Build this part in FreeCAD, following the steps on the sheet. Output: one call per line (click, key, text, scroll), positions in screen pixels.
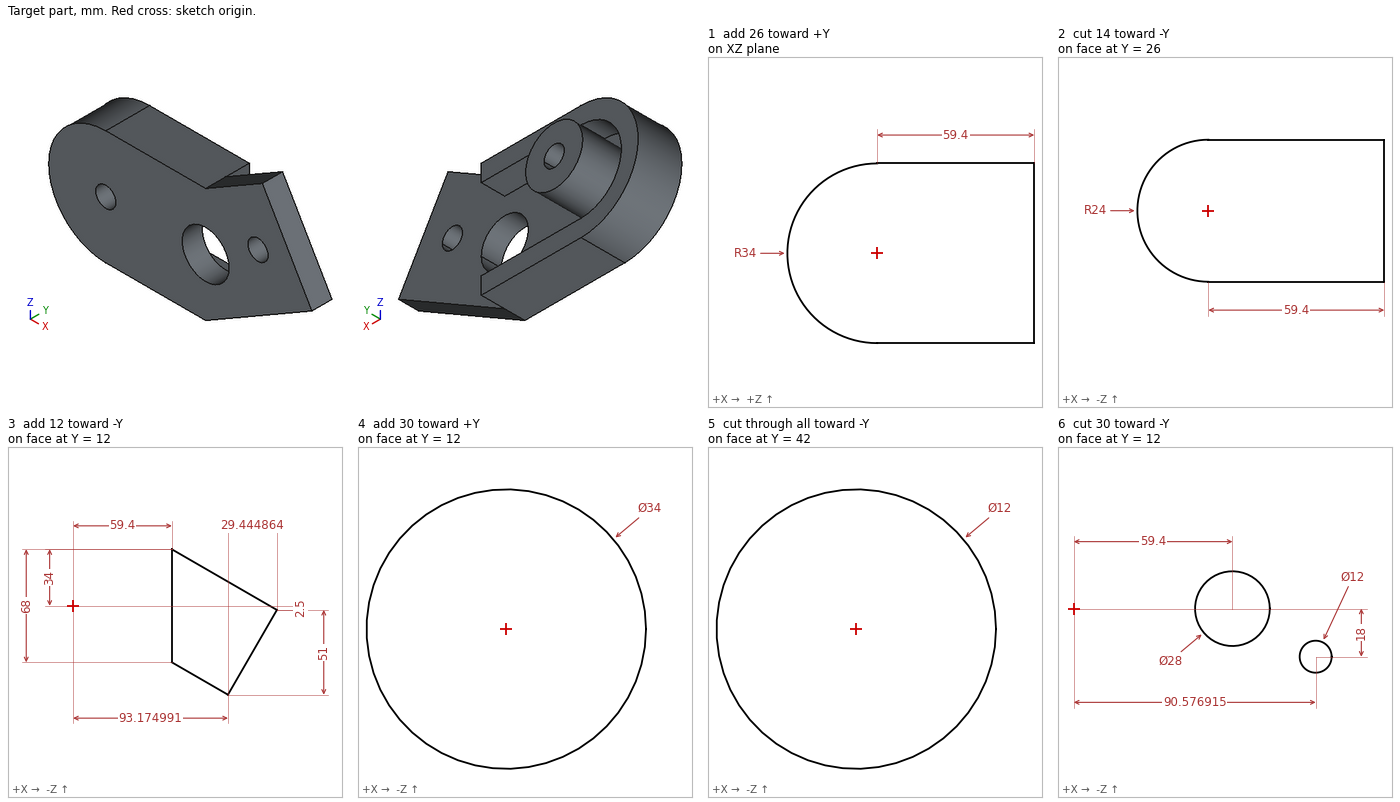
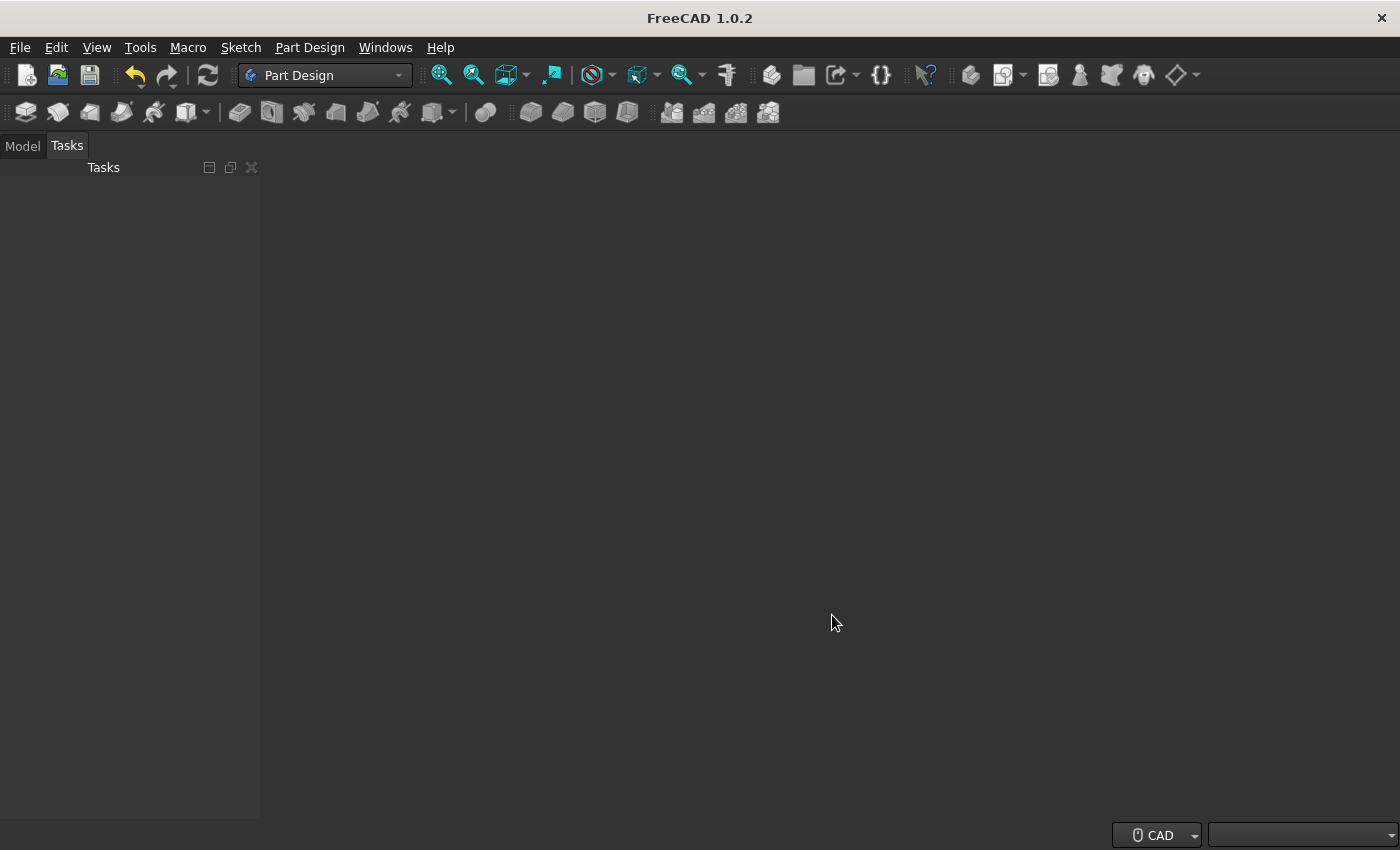
click(26, 76)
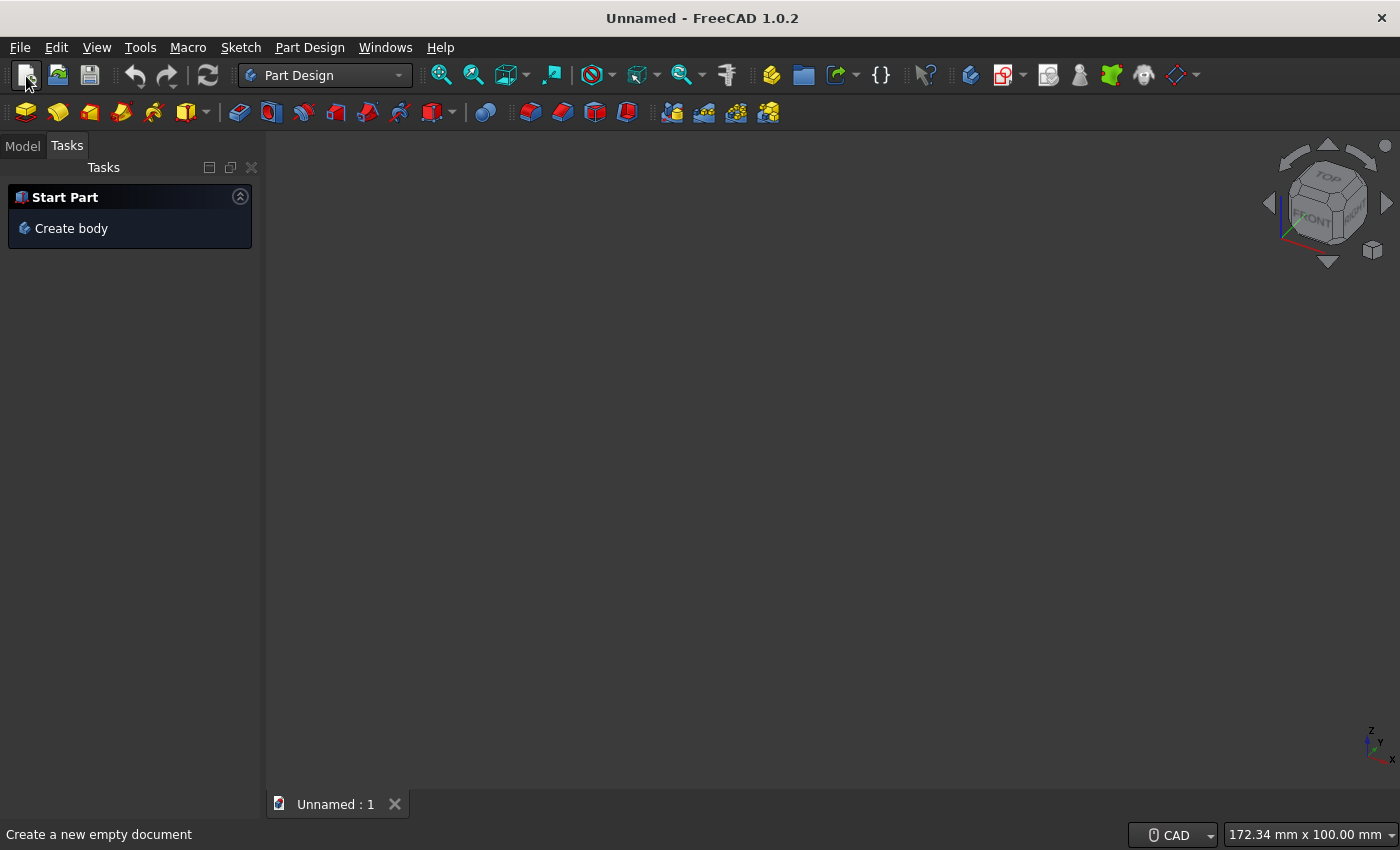
click(1004, 76)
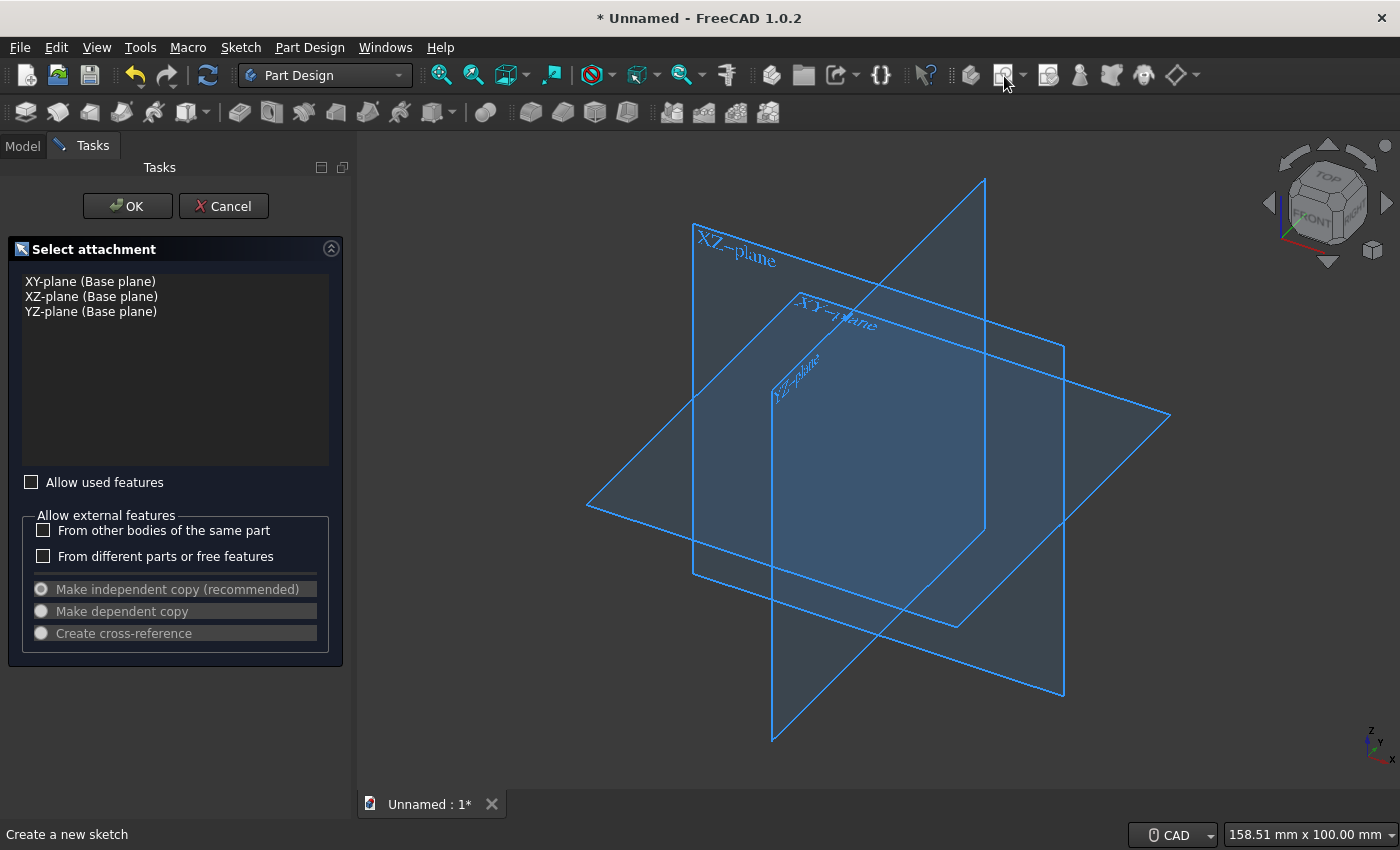
click(82, 296)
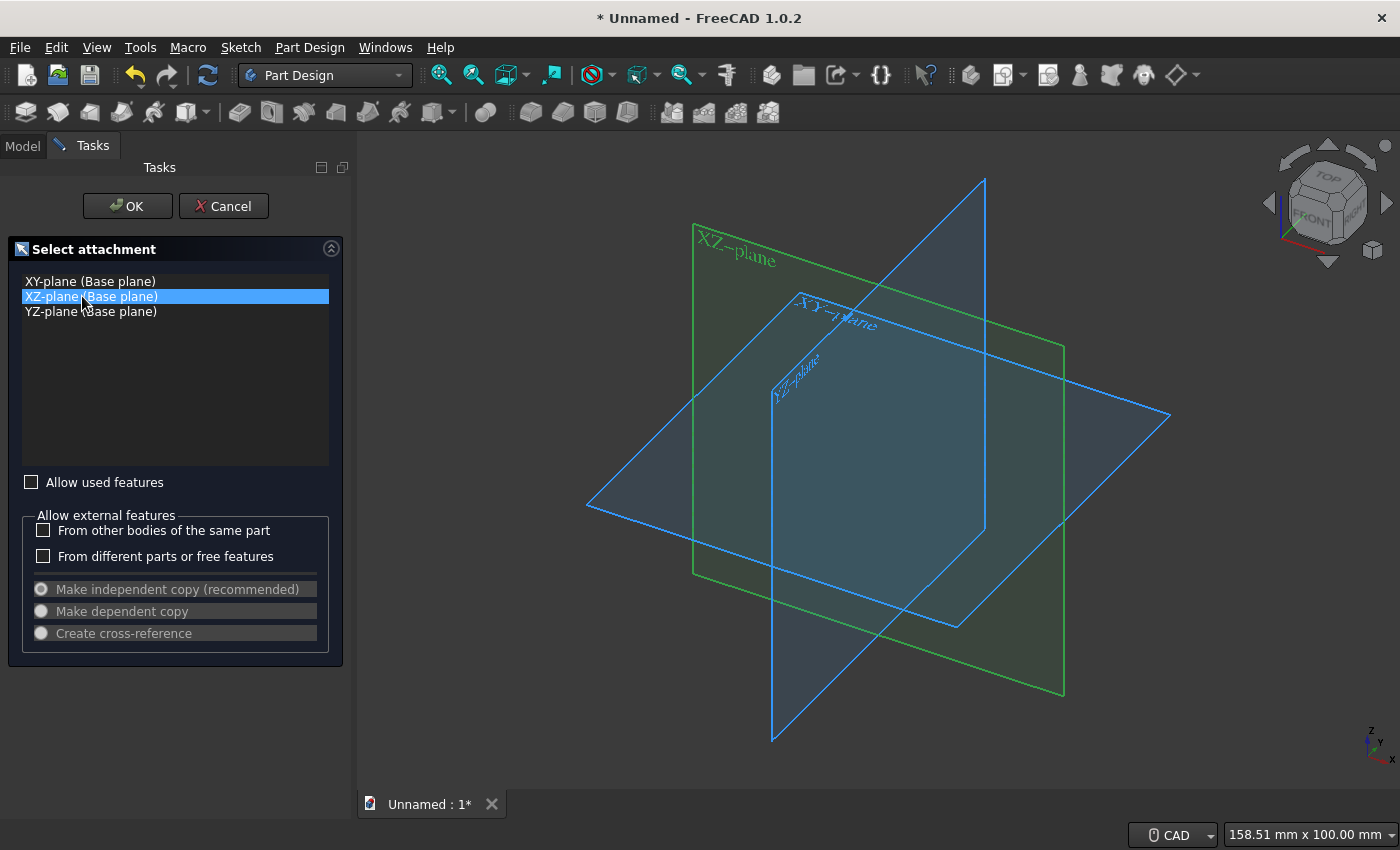
click(128, 206)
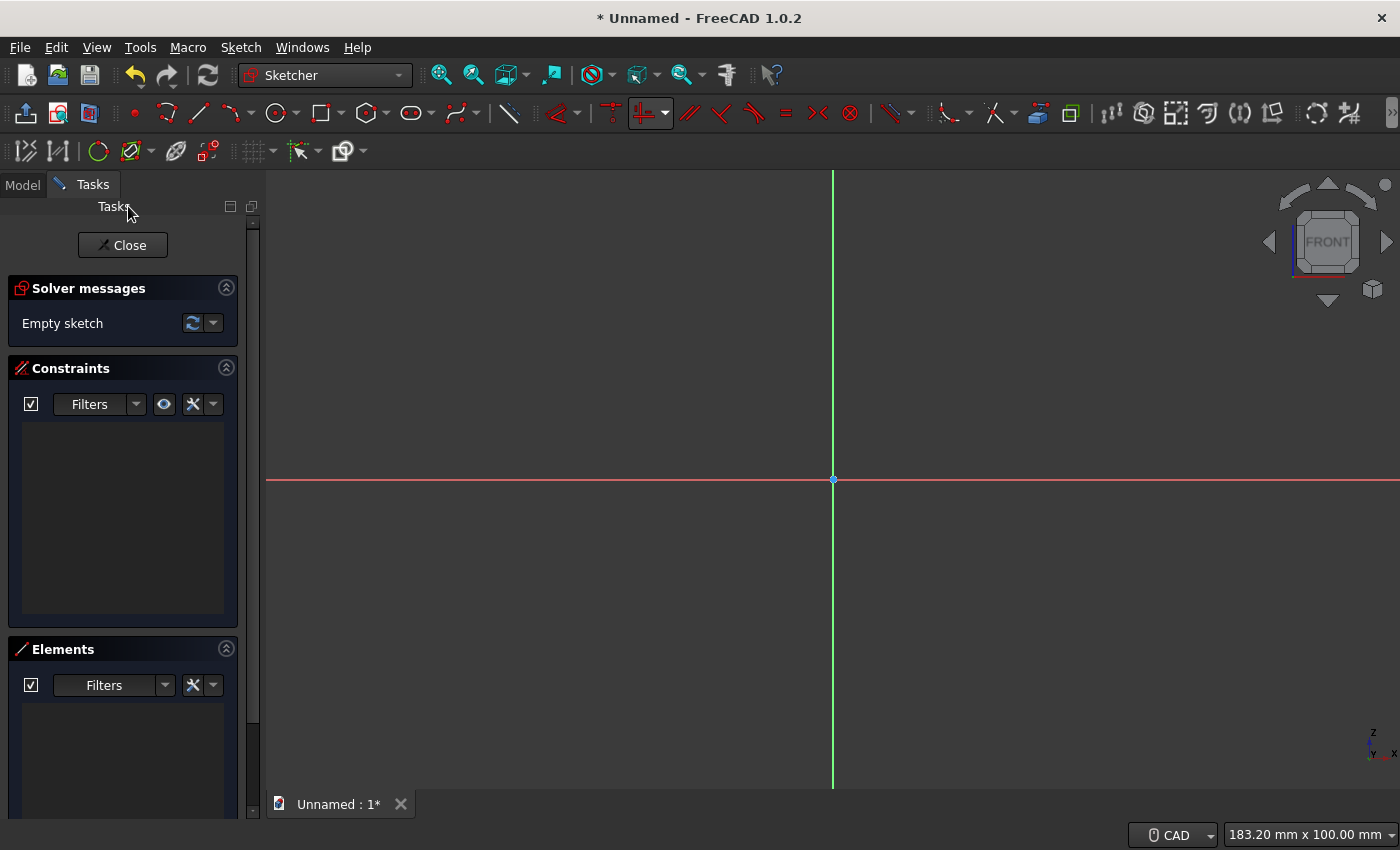
click(168, 114)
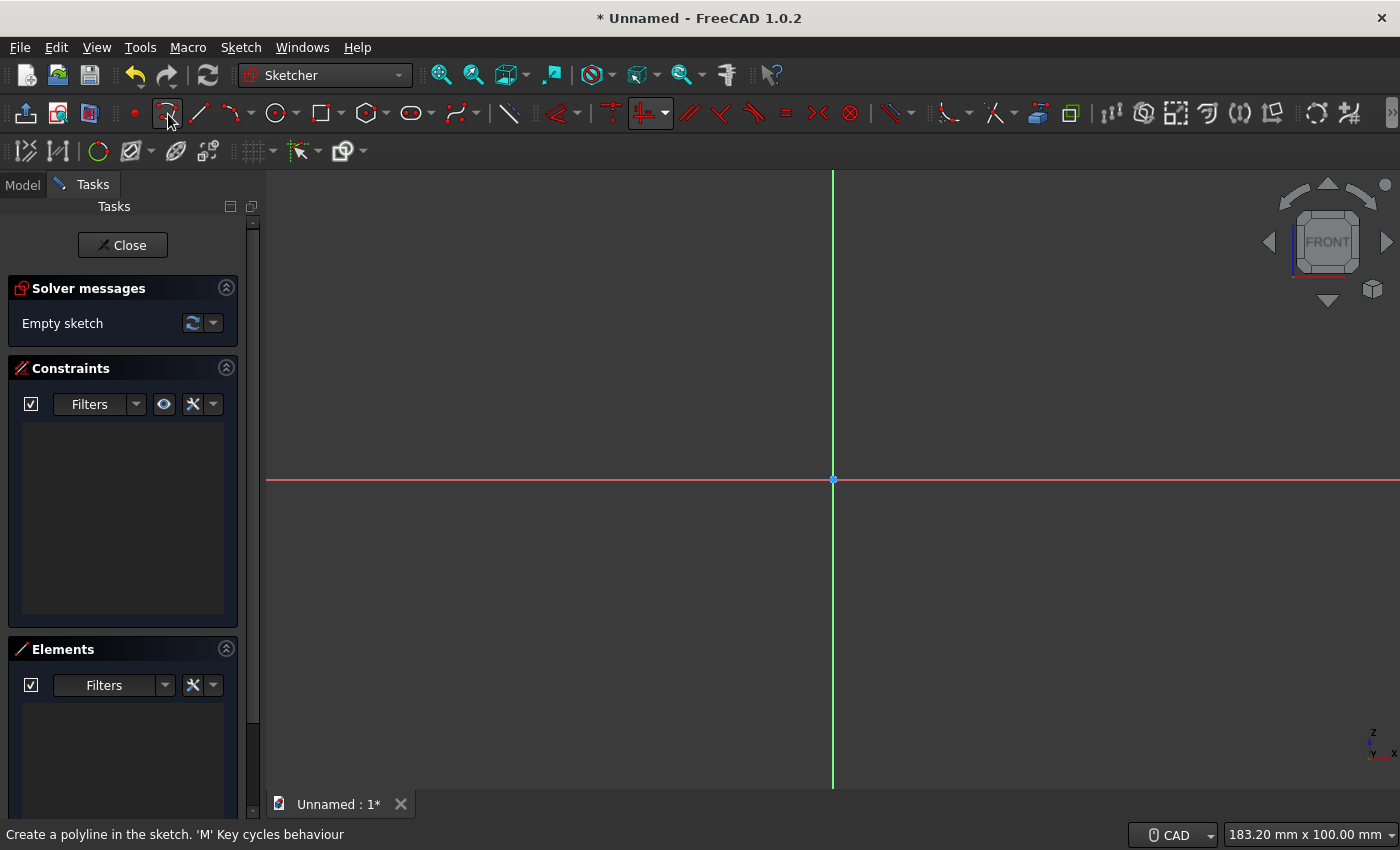
click(833, 269)
click(1201, 269)
click(1201, 690)
click(833, 690)
right_click(833, 690)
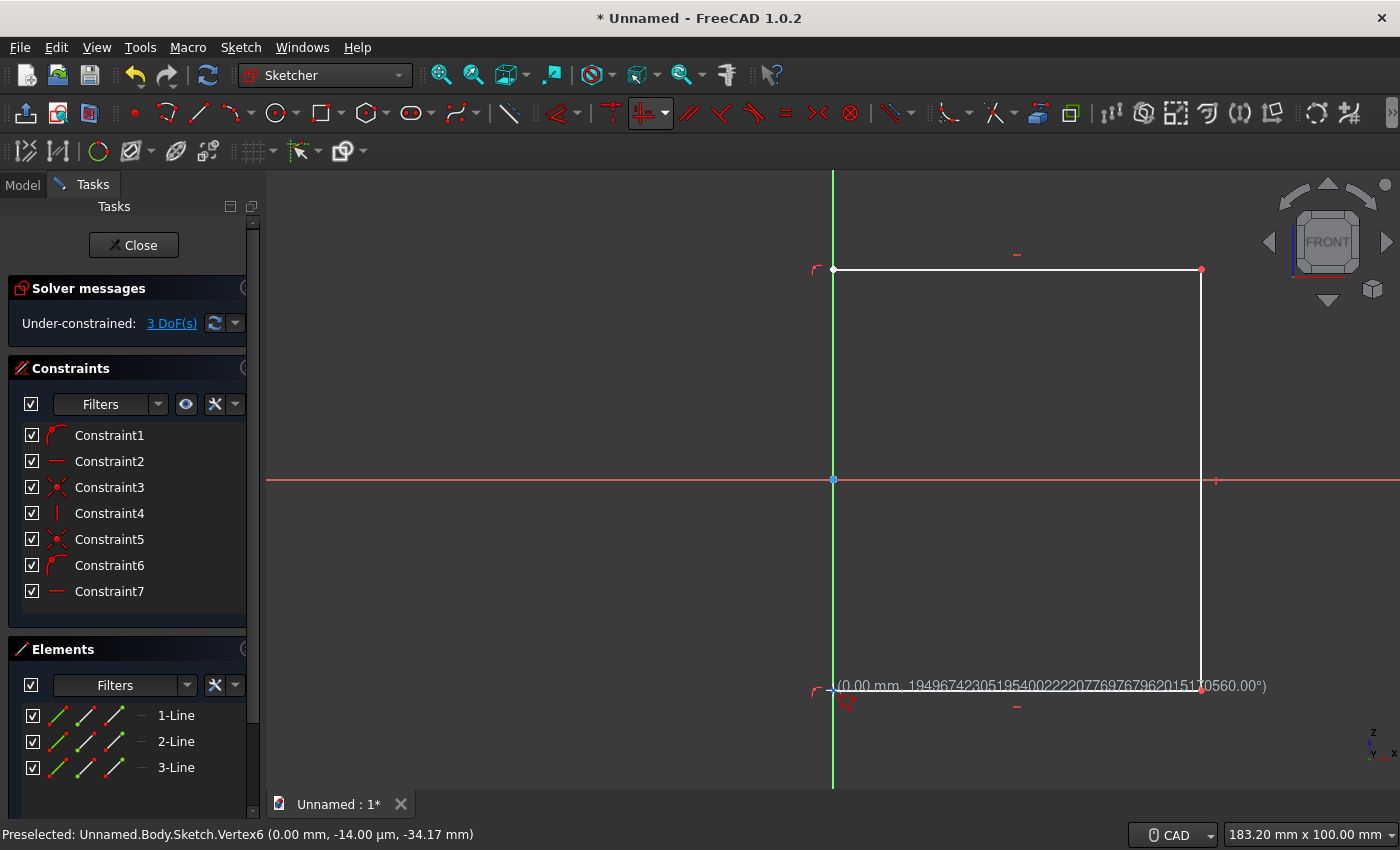
click(232, 114)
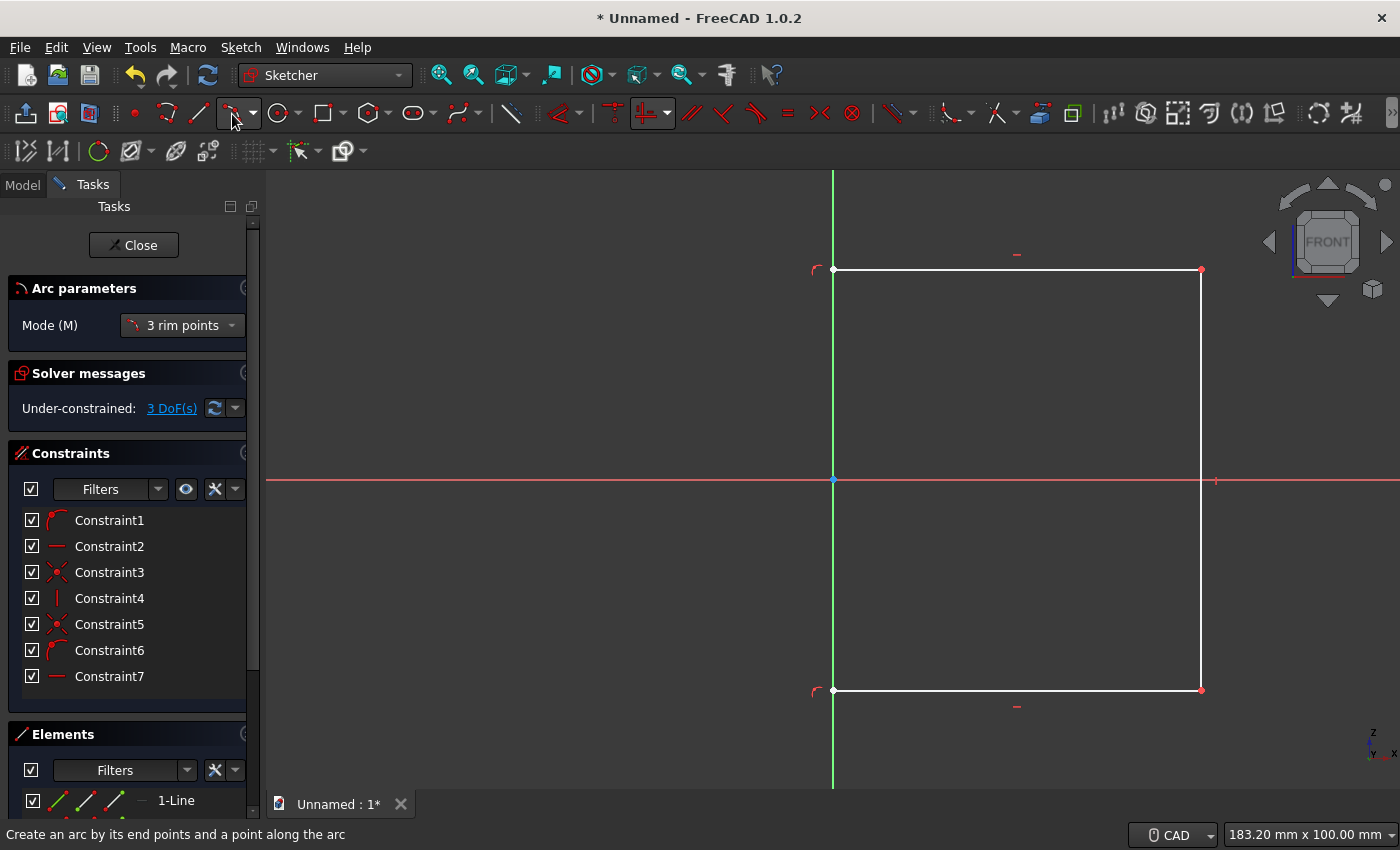
click(833, 691)
click(833, 270)
click(633, 414)
key(Escape)